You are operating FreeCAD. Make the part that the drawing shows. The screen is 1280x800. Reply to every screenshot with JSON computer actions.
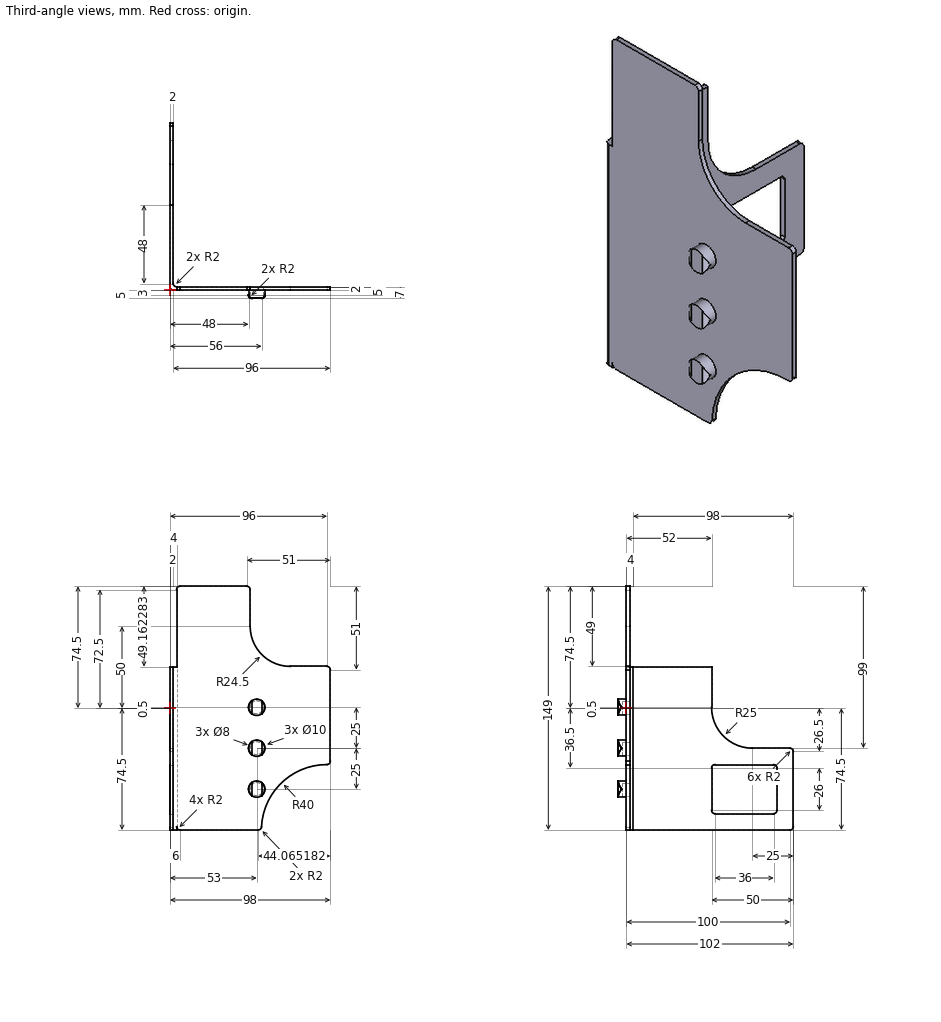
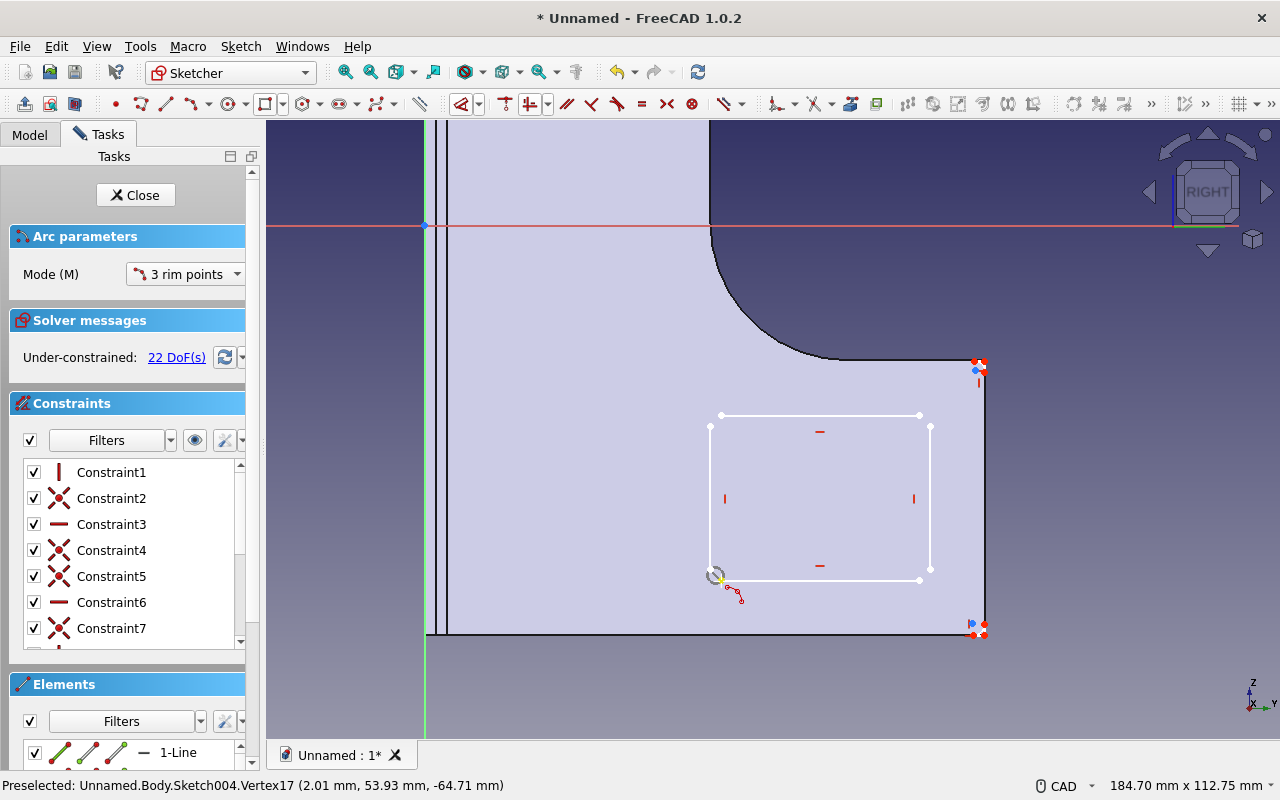
{"action": "scroll", "coordinate": [714, 577], "scroll_direction": "up", "scroll_amount": 8}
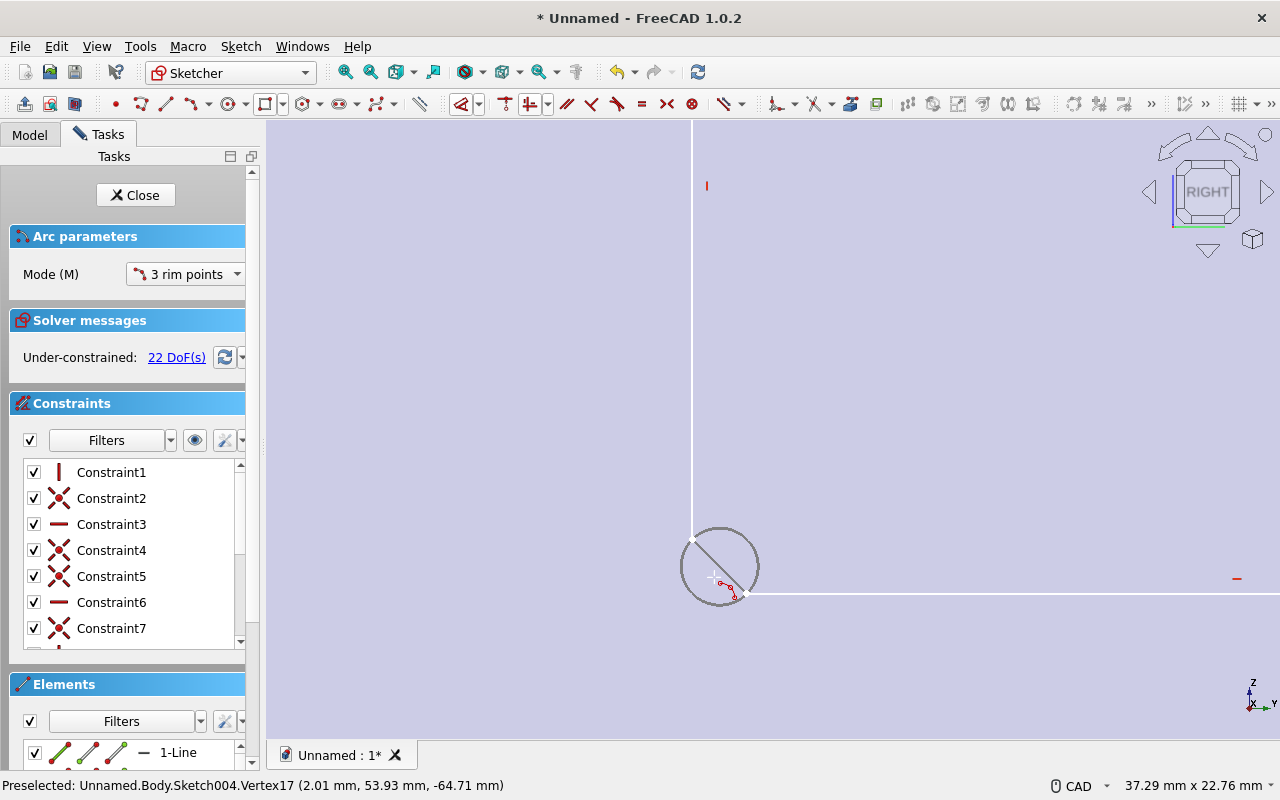
{"action": "left_click", "coordinate": [710, 572]}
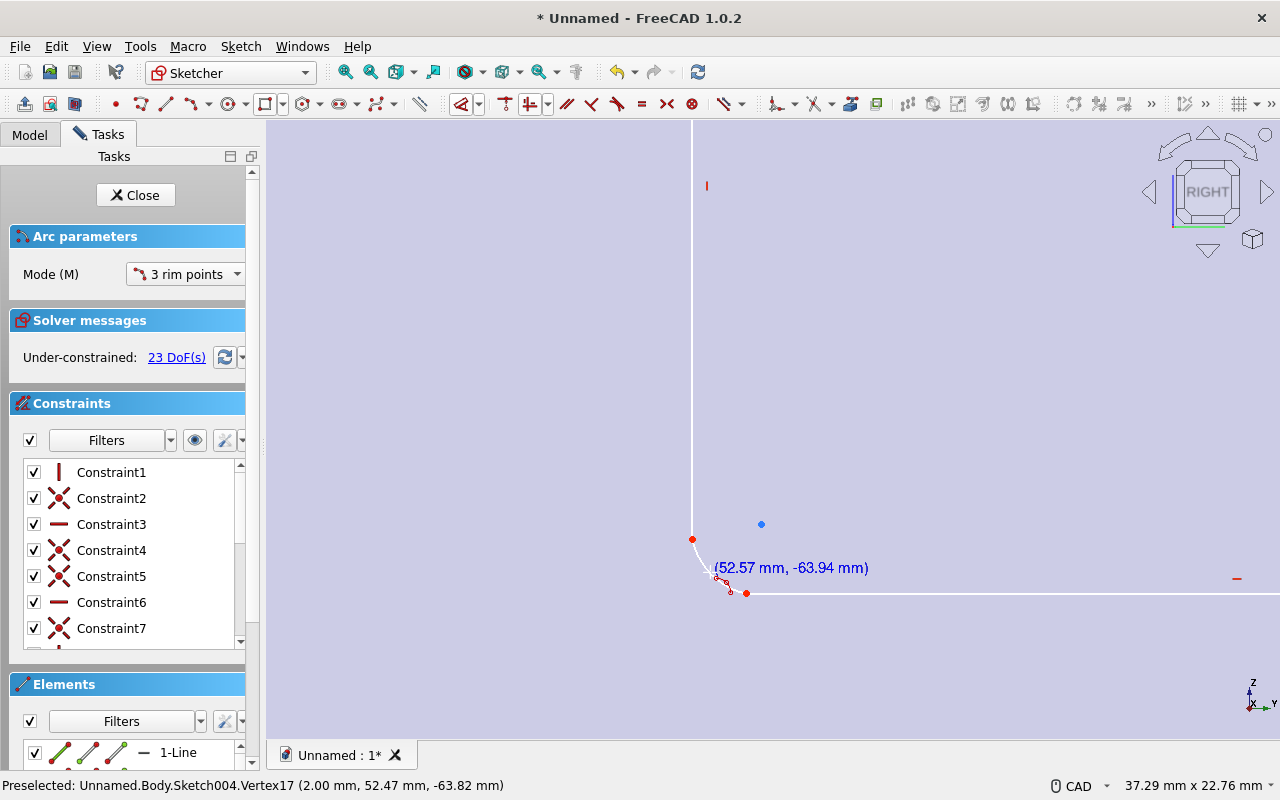
{"action": "scroll", "coordinate": [714, 577], "scroll_direction": "down", "scroll_amount": 8}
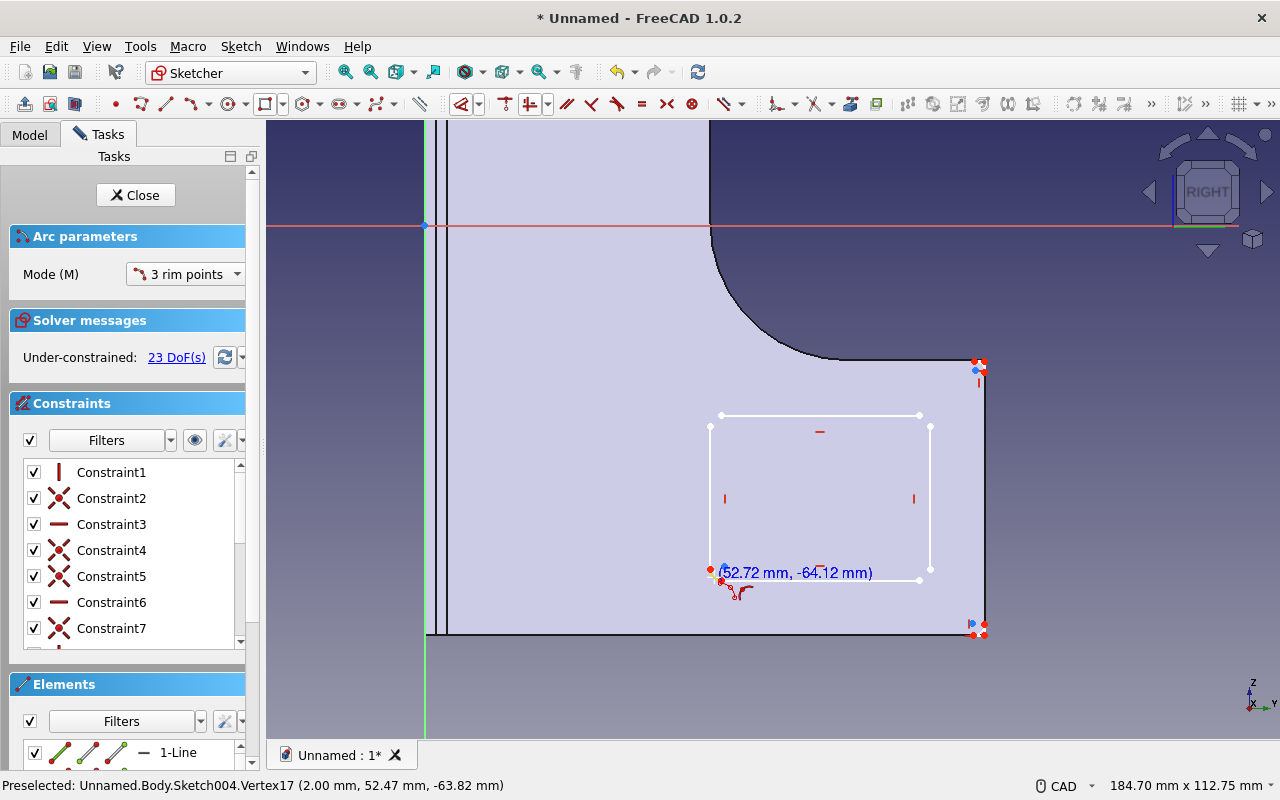
{"action": "left_click", "coordinate": [919, 581]}
{"action": "left_click", "coordinate": [930, 570]}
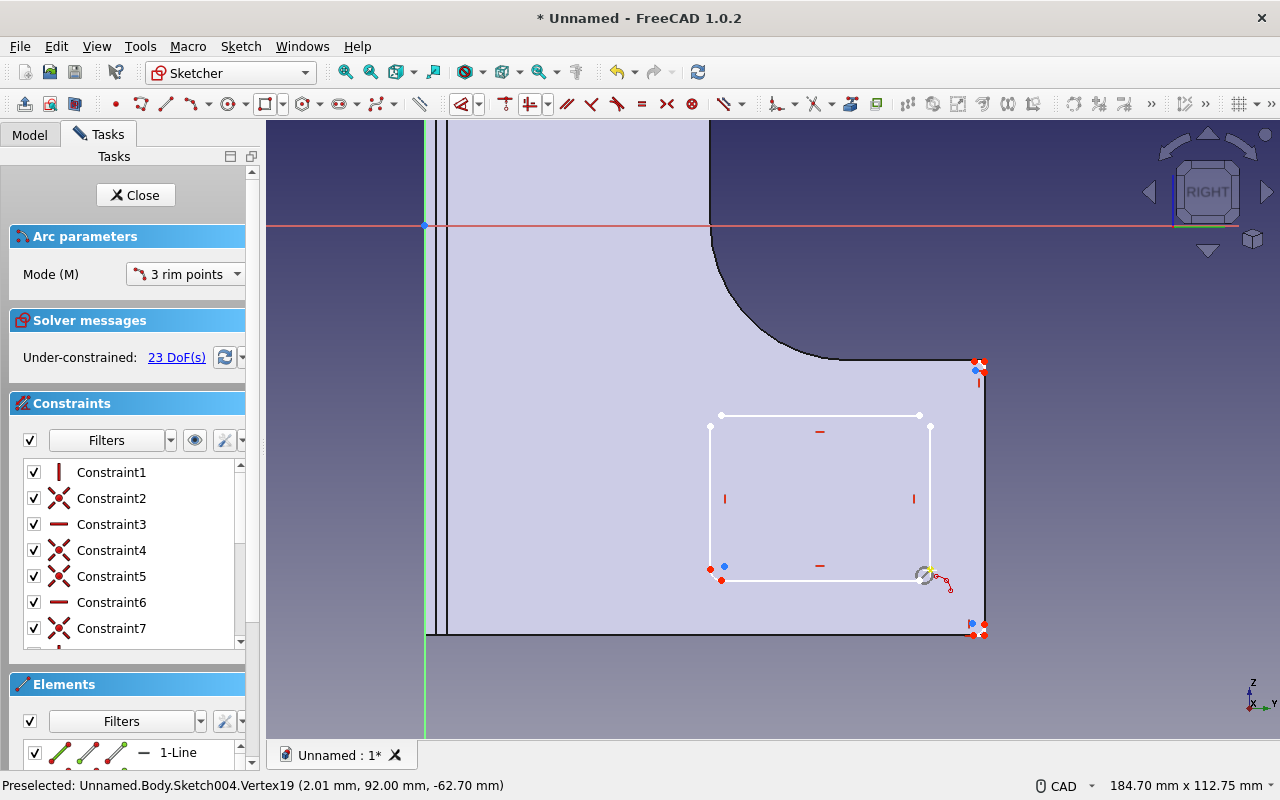
{"action": "scroll", "coordinate": [927, 577], "scroll_direction": "up", "scroll_amount": 8}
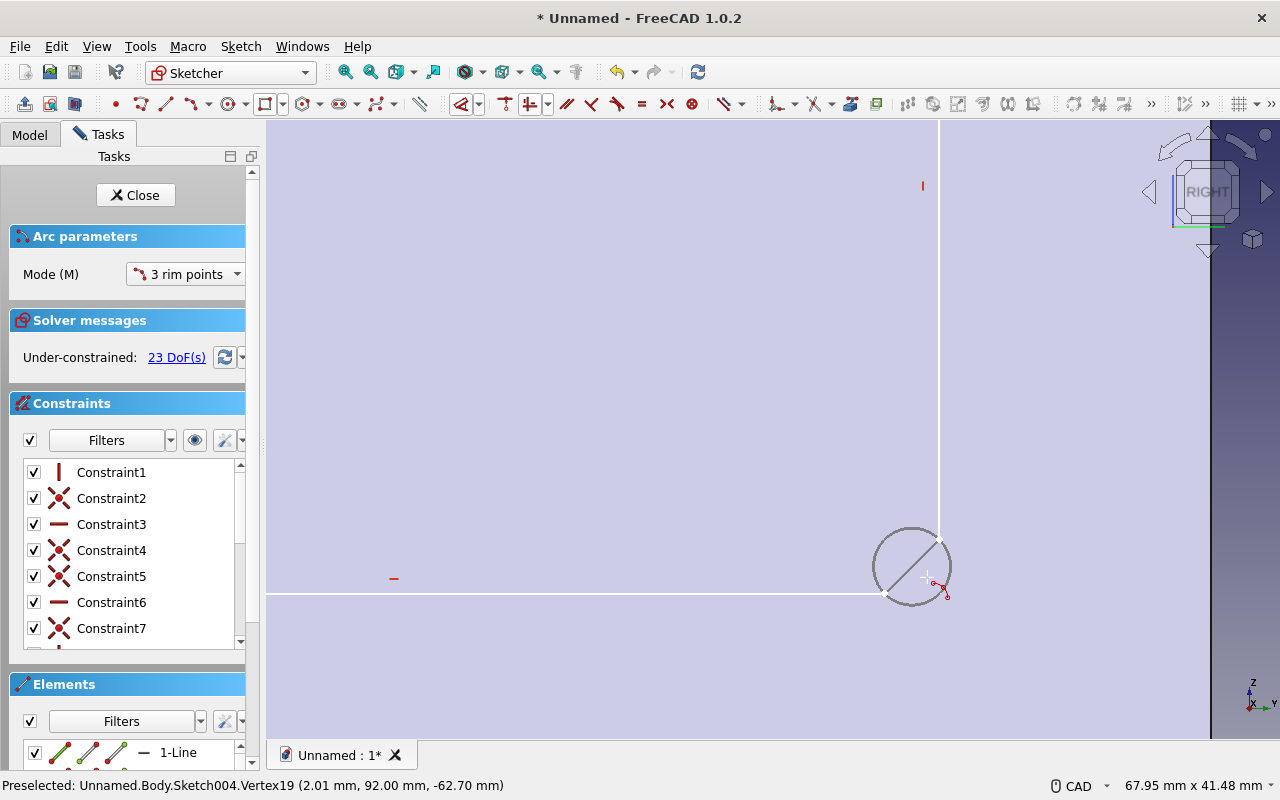
{"action": "left_click", "coordinate": [923, 572]}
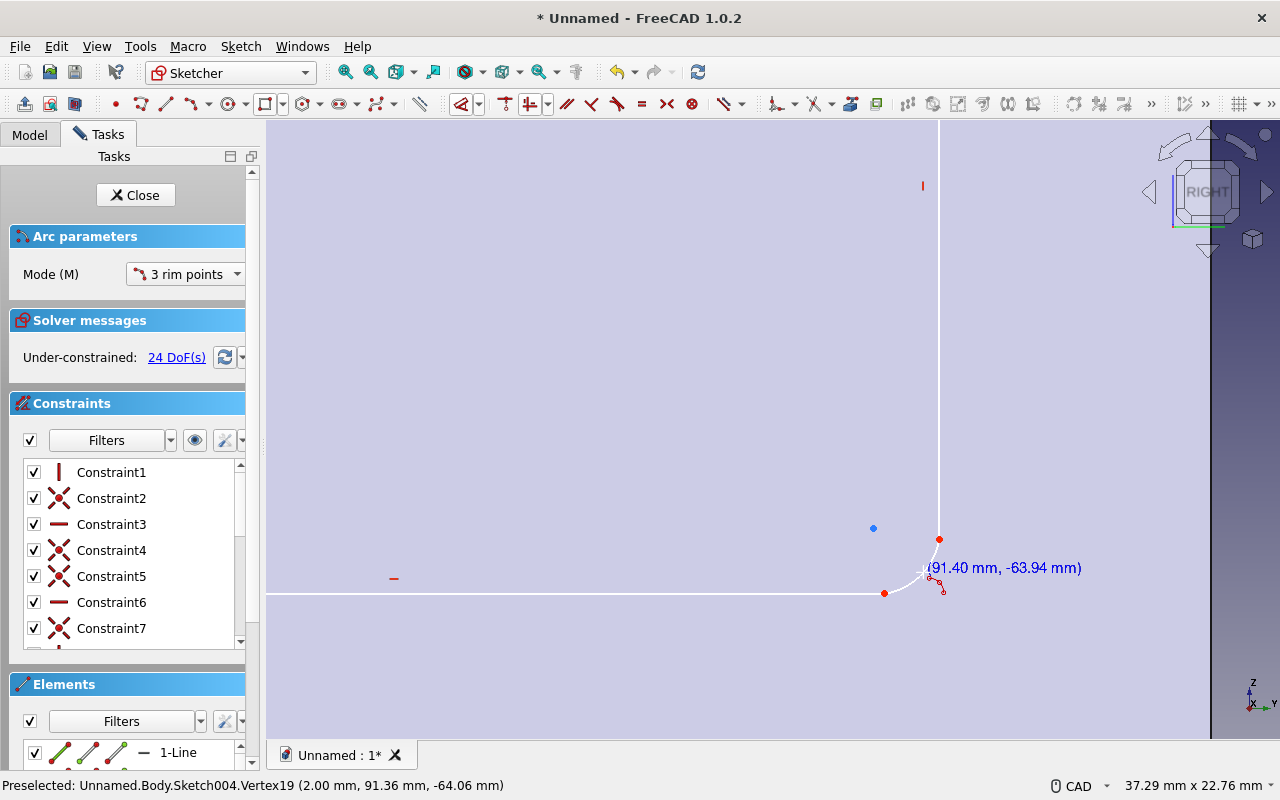
{"action": "scroll", "coordinate": [927, 577], "scroll_direction": "down", "scroll_amount": 8}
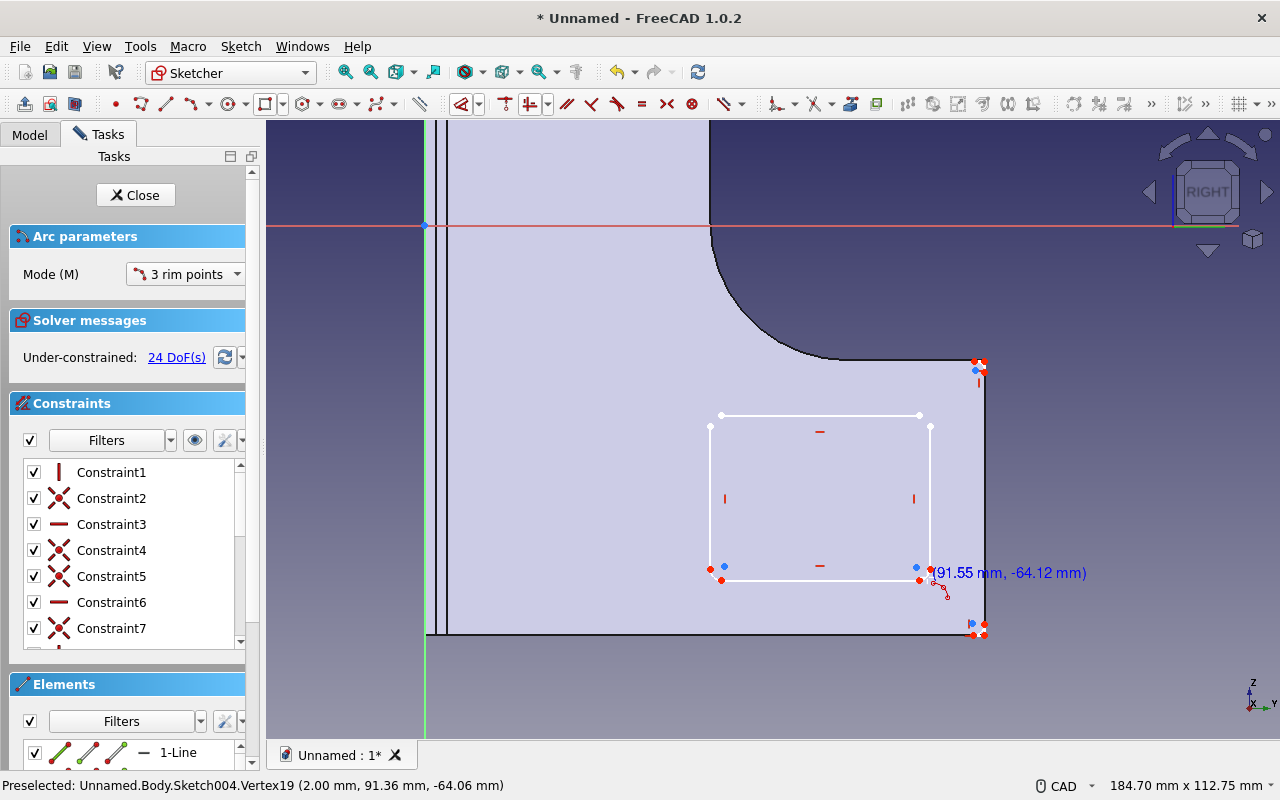
{"action": "left_click", "coordinate": [930, 427]}
{"action": "left_click", "coordinate": [919, 416]}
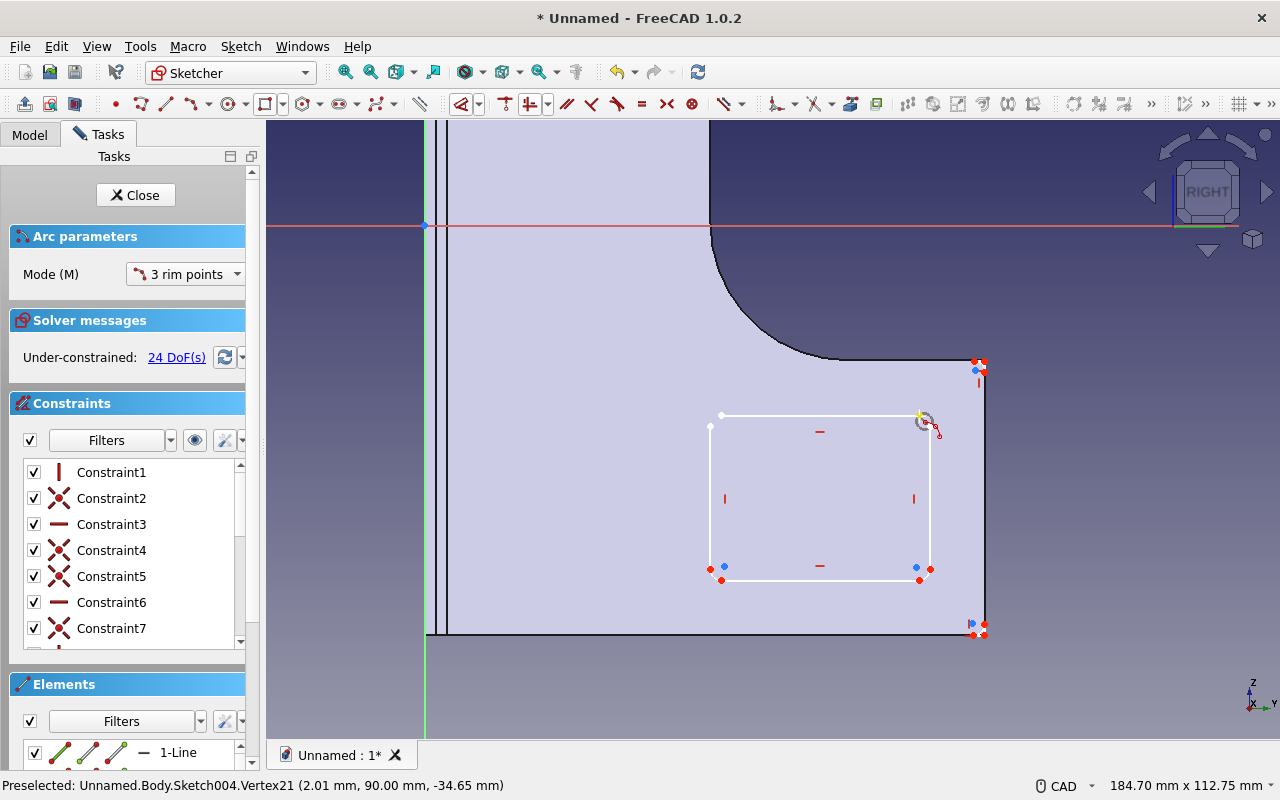
{"action": "scroll", "coordinate": [927, 418], "scroll_direction": "up", "scroll_amount": 8}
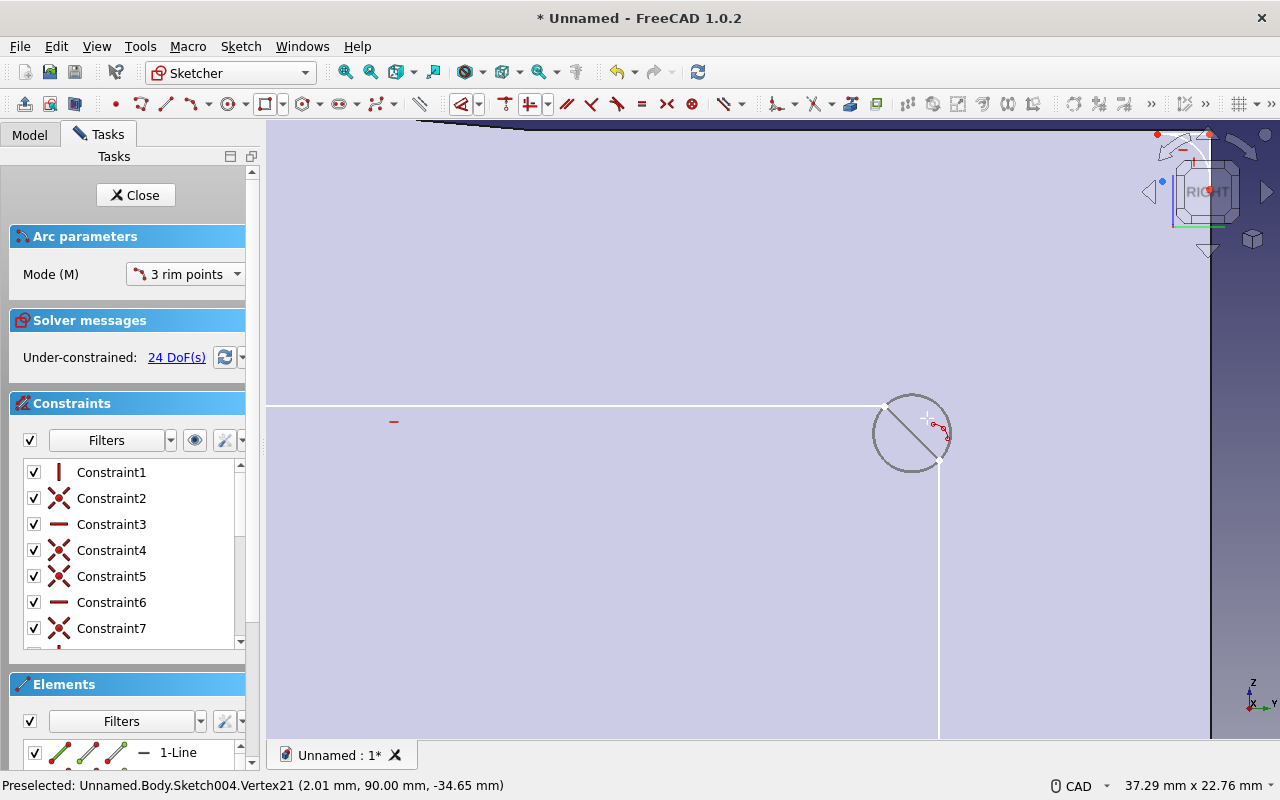
{"action": "left_click", "coordinate": [923, 418]}